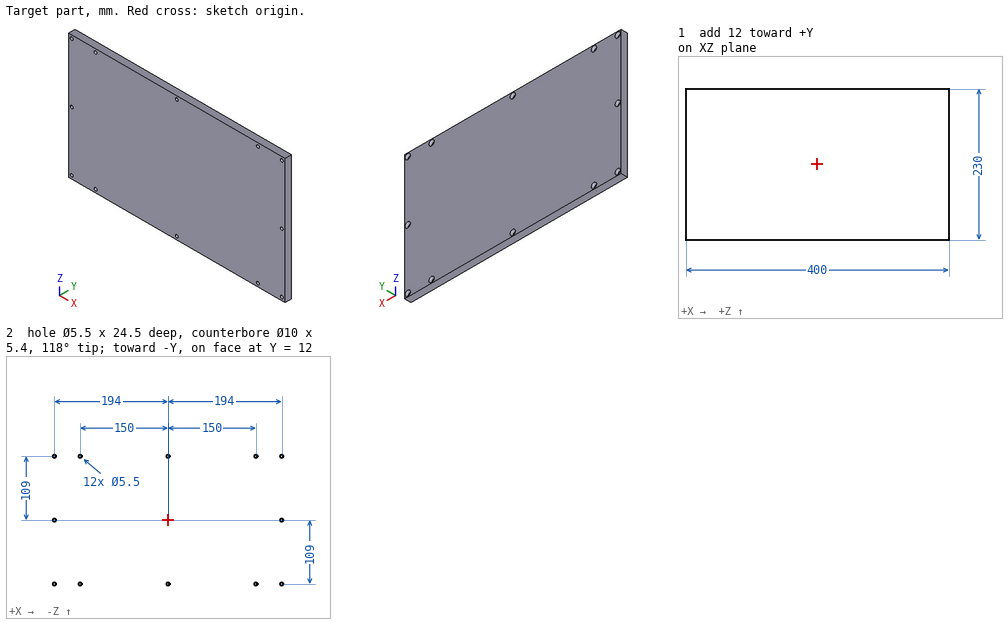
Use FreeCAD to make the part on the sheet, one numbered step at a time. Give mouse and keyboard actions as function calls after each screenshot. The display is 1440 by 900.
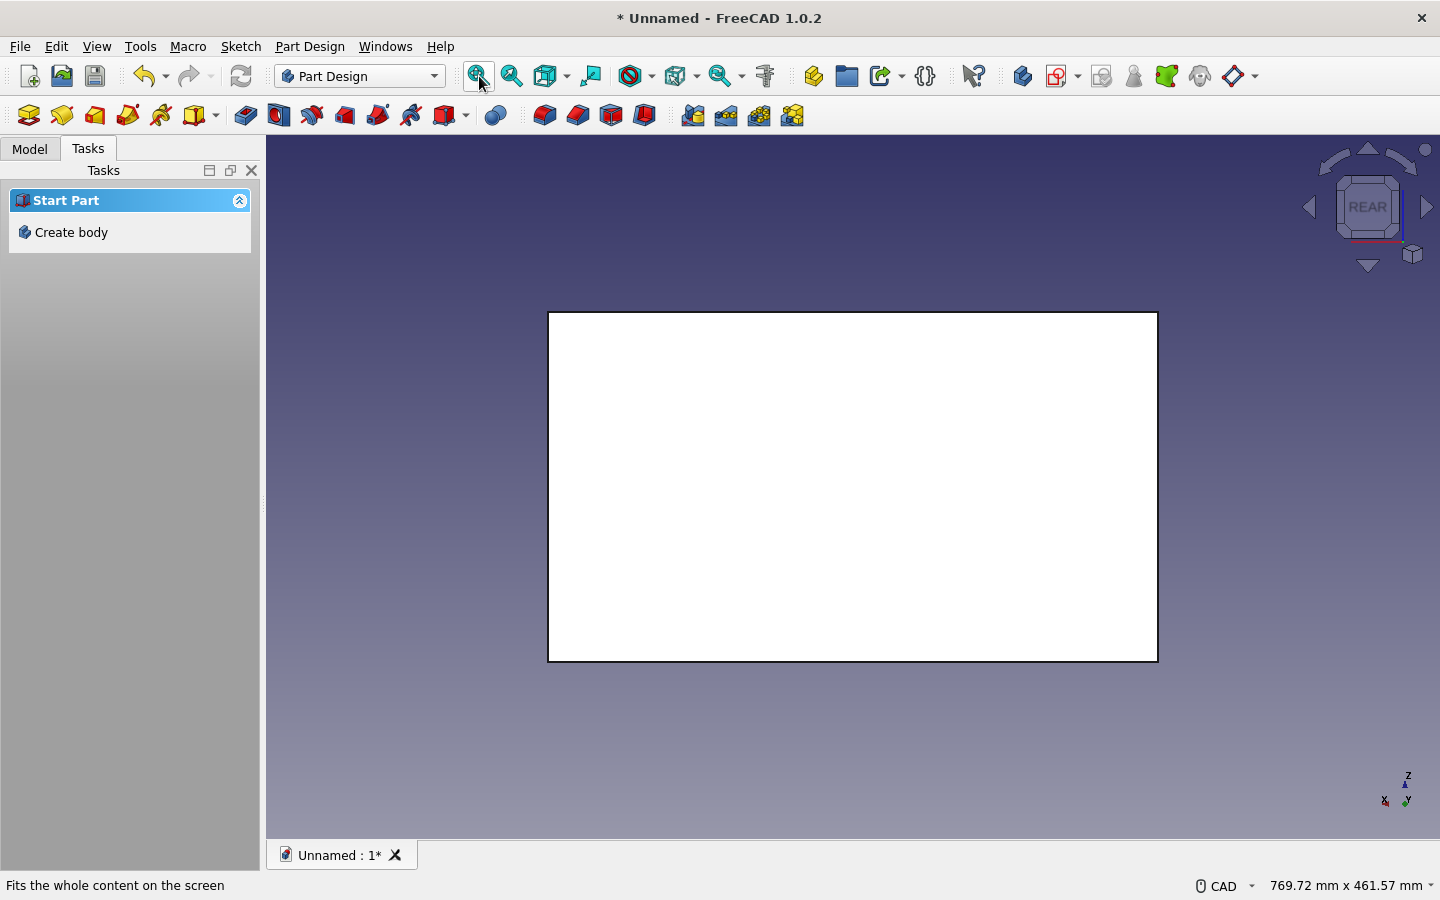
click(766, 486)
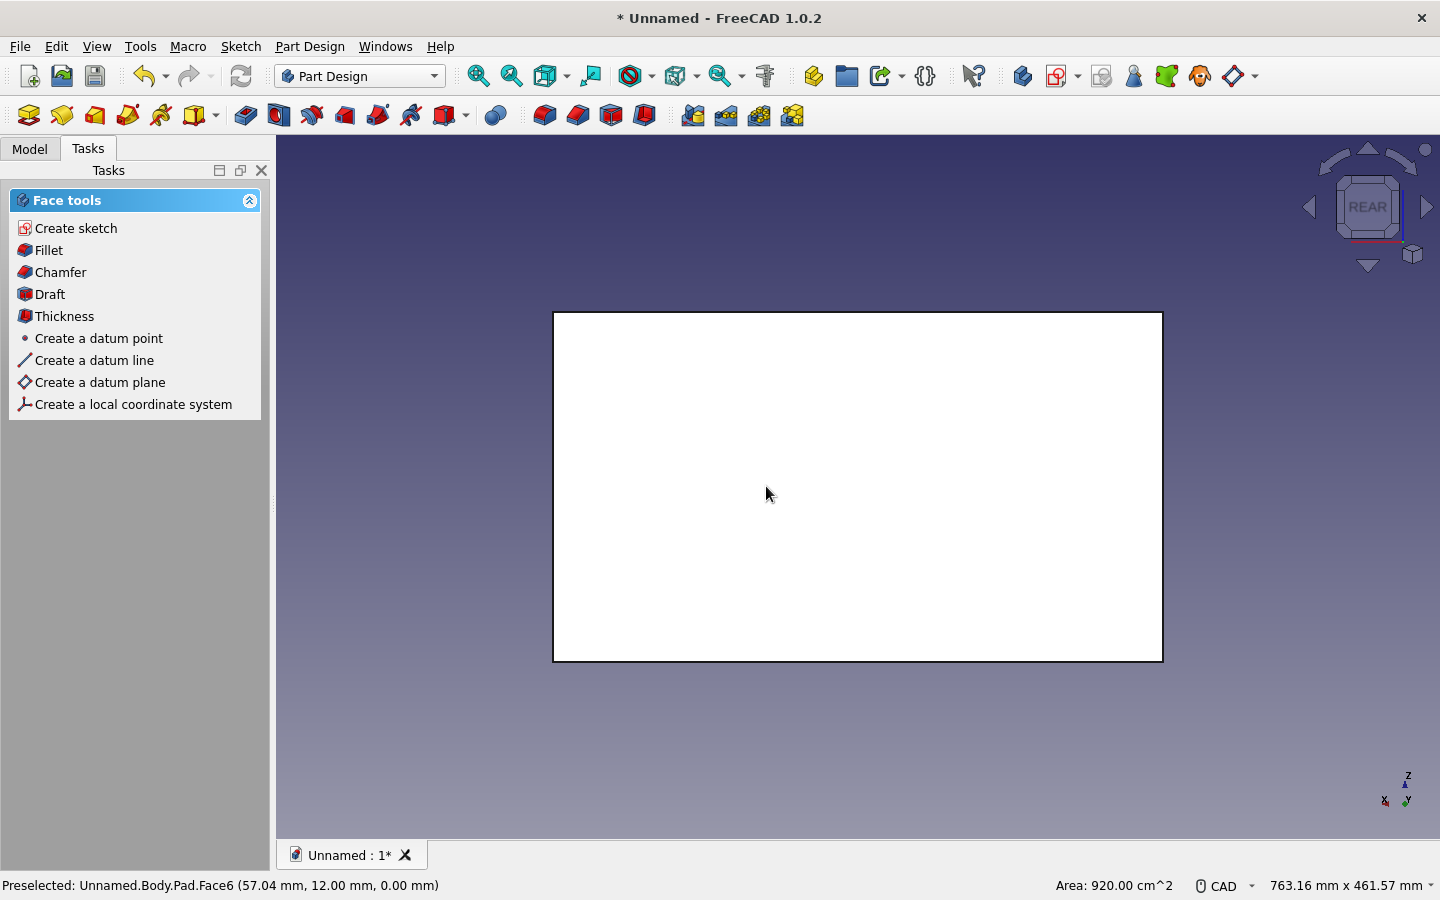
click(1056, 76)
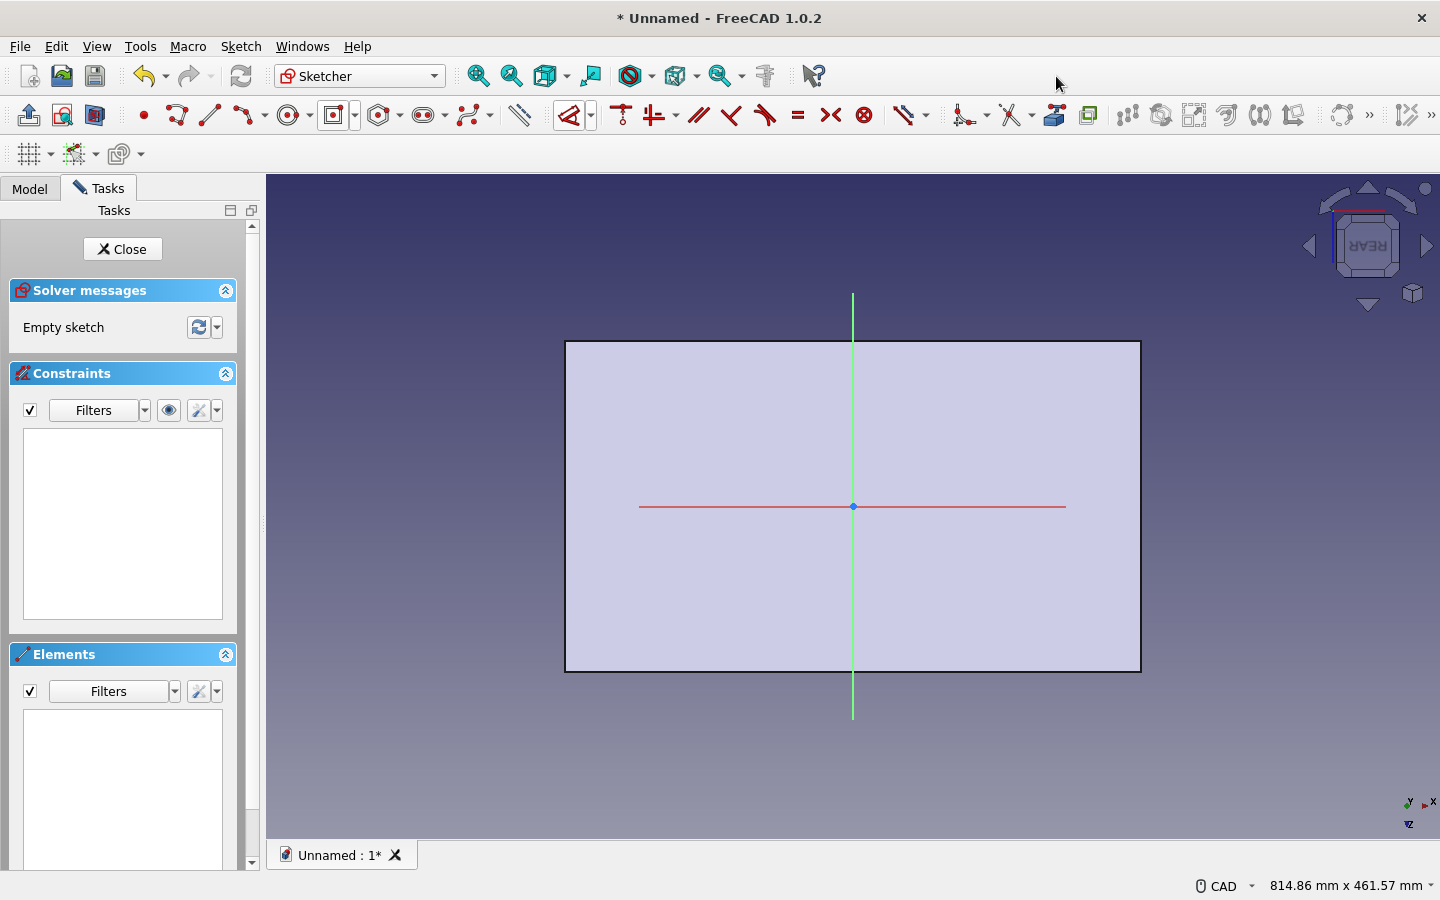
click(288, 116)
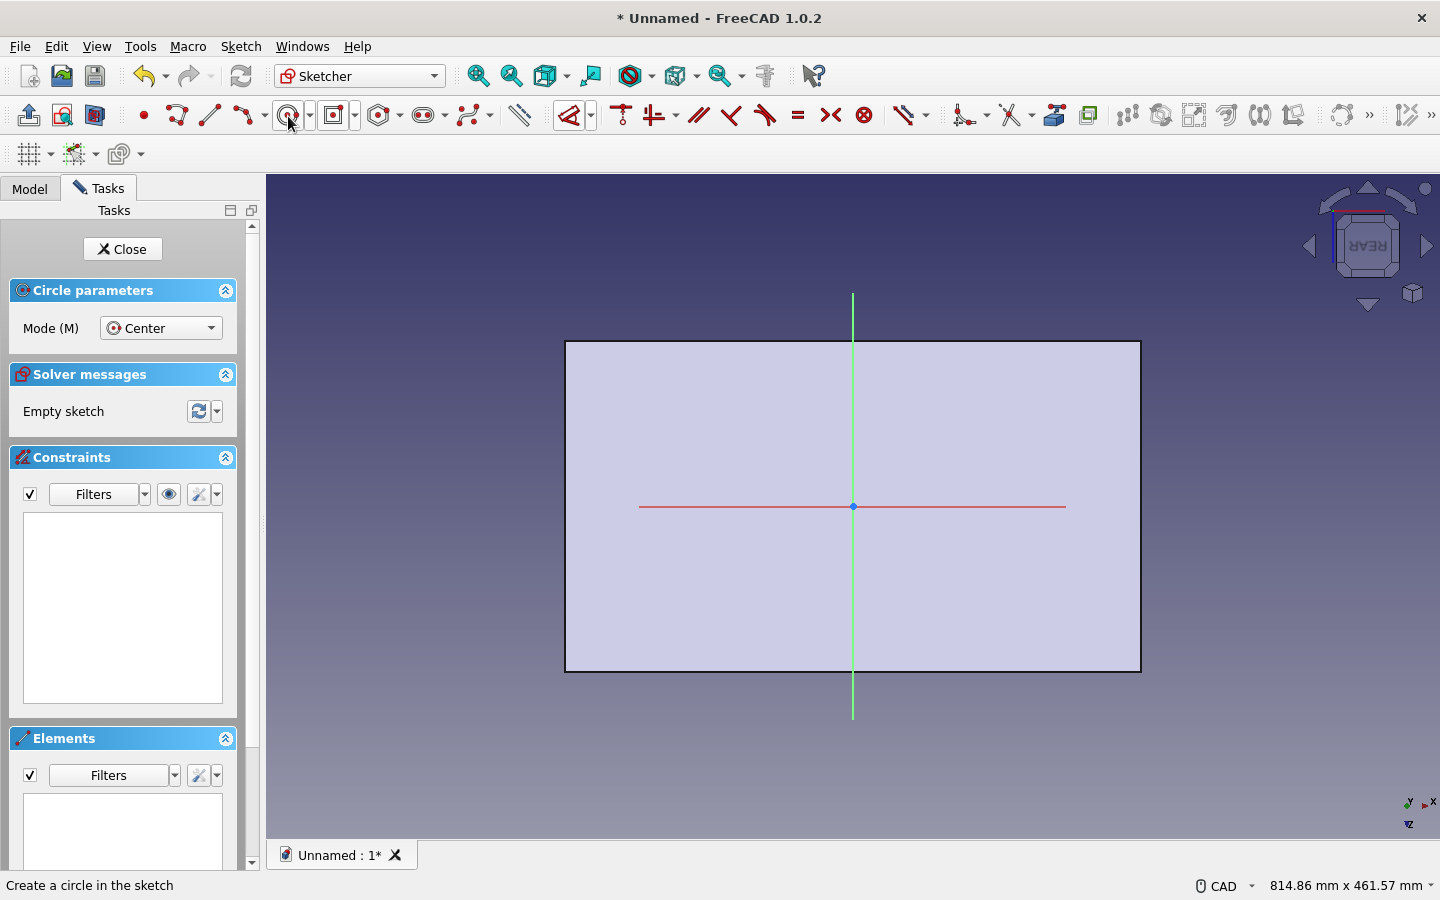
scroll(573, 349, up, 9)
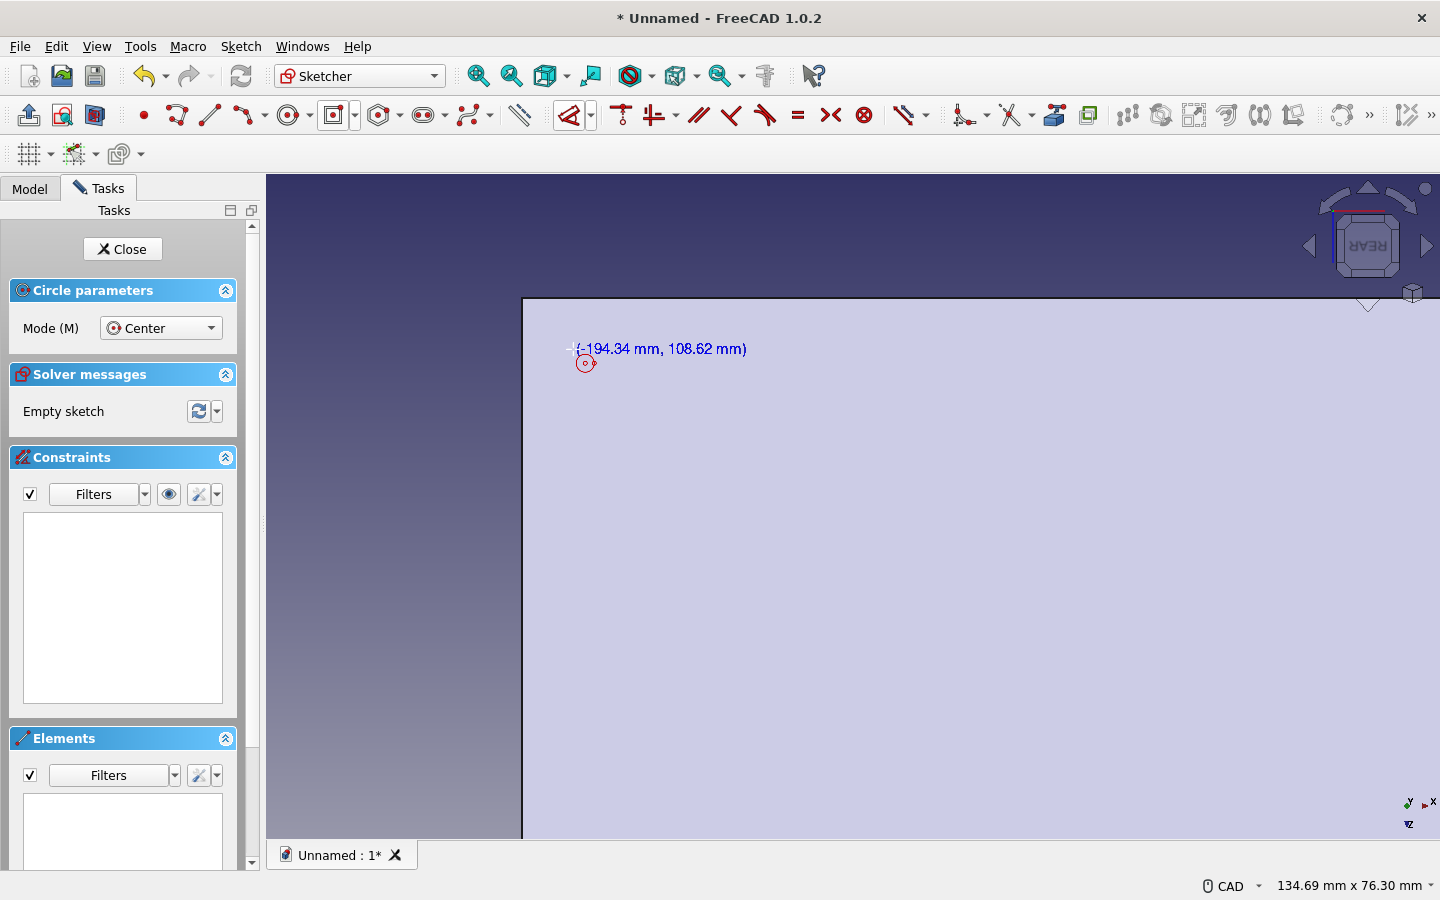
scroll(410, 306, down, 8)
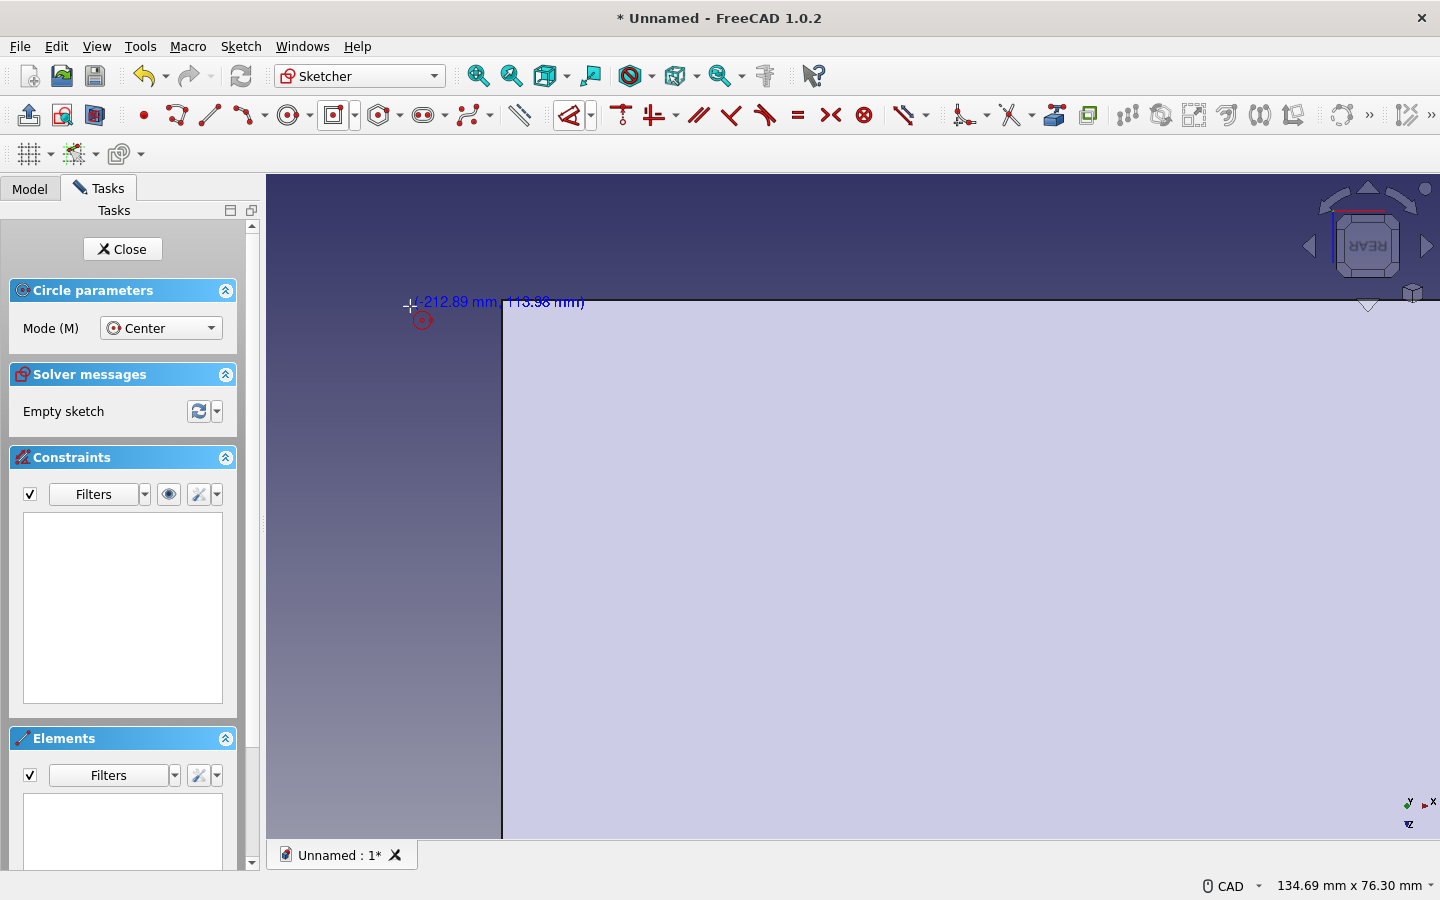
click(443, 315)
move(447, 312)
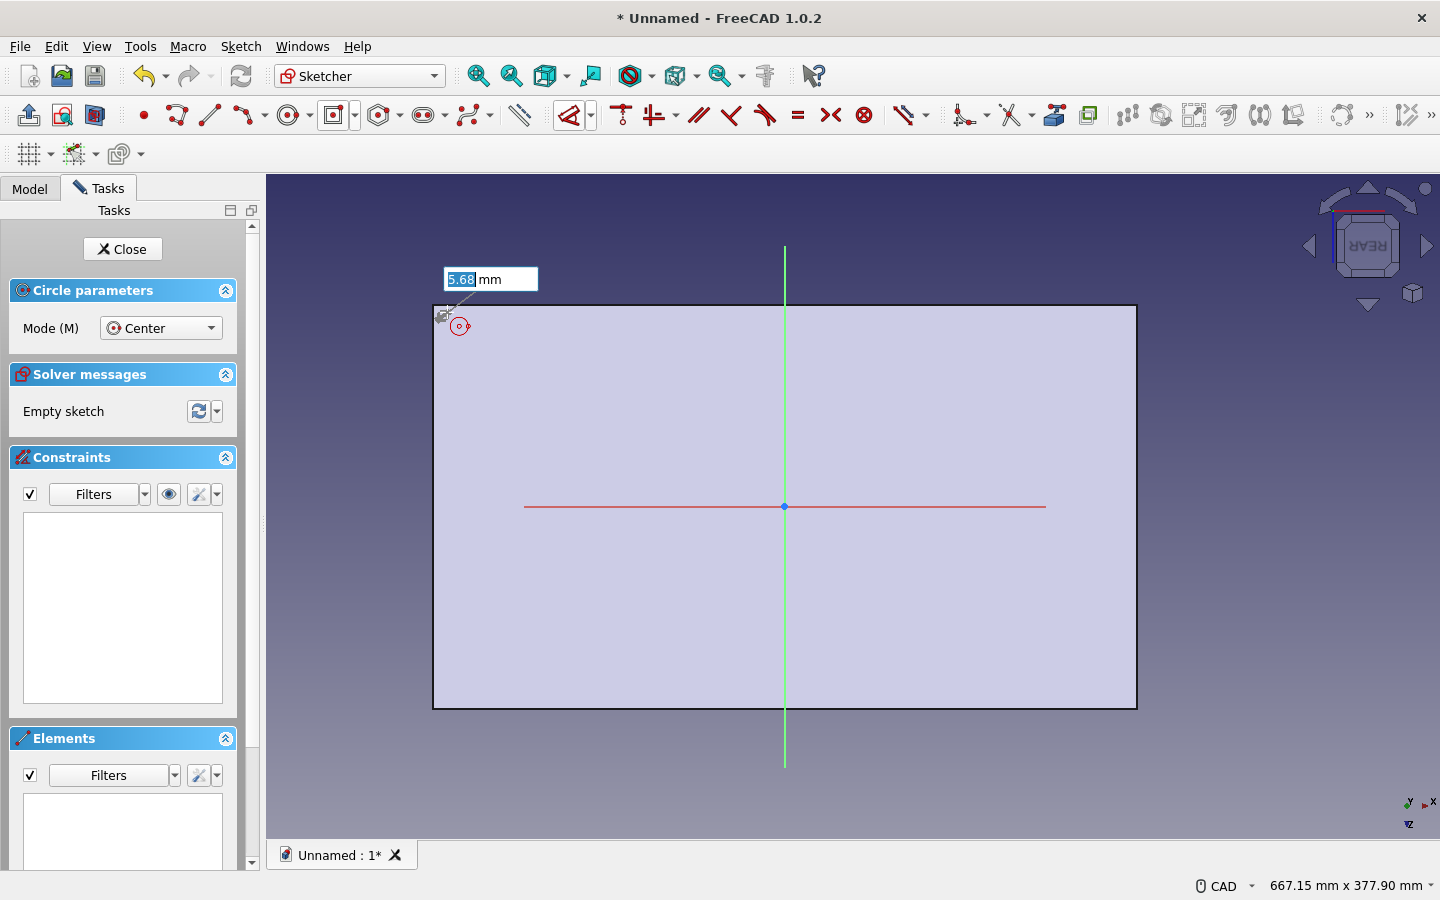
text(5.5)
key(Return)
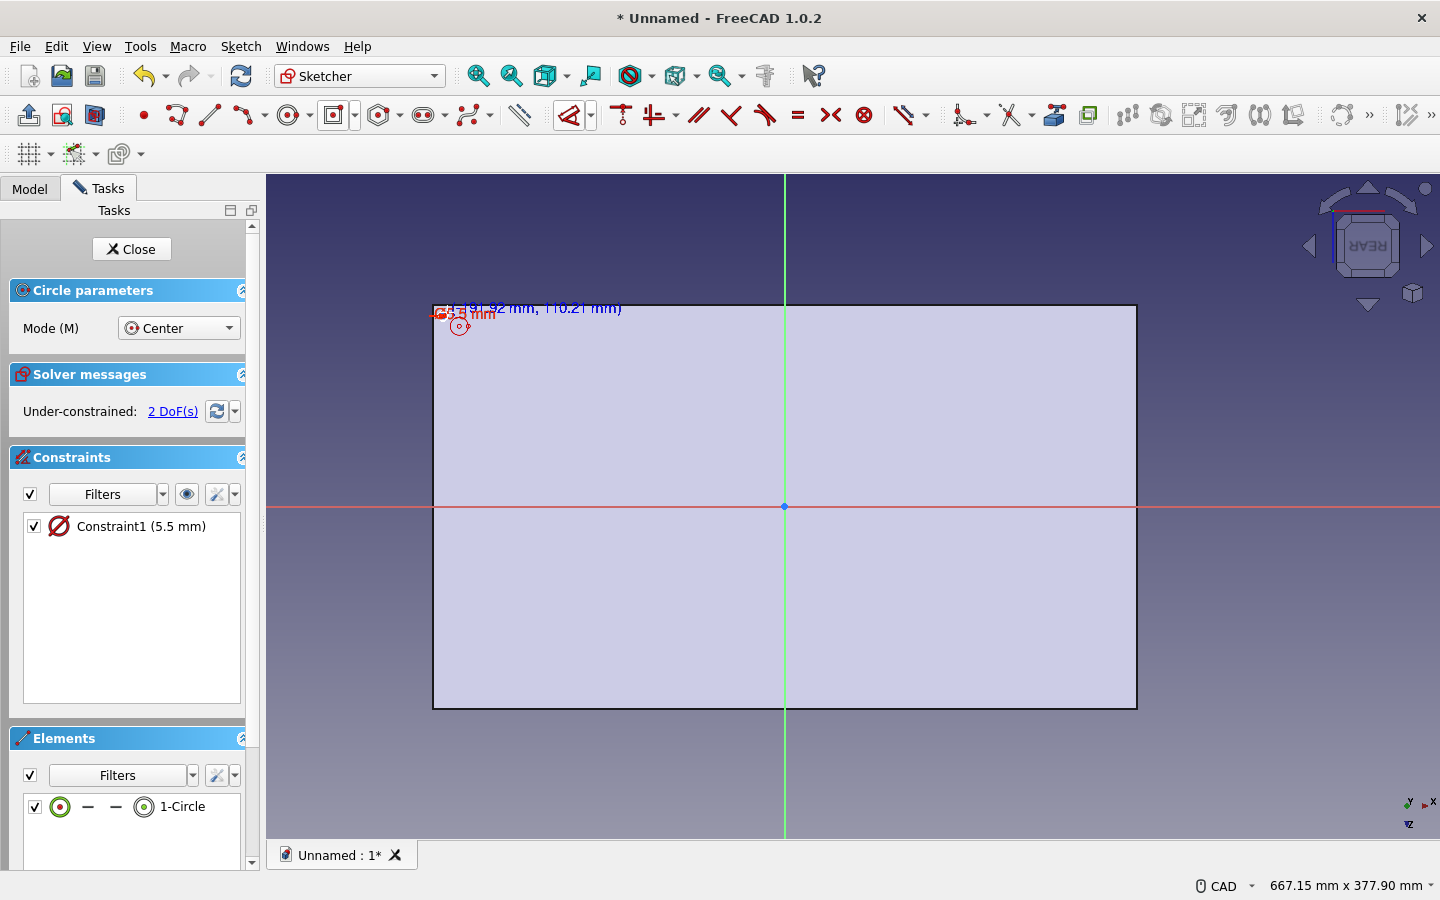
scroll(521, 315, up, 8)